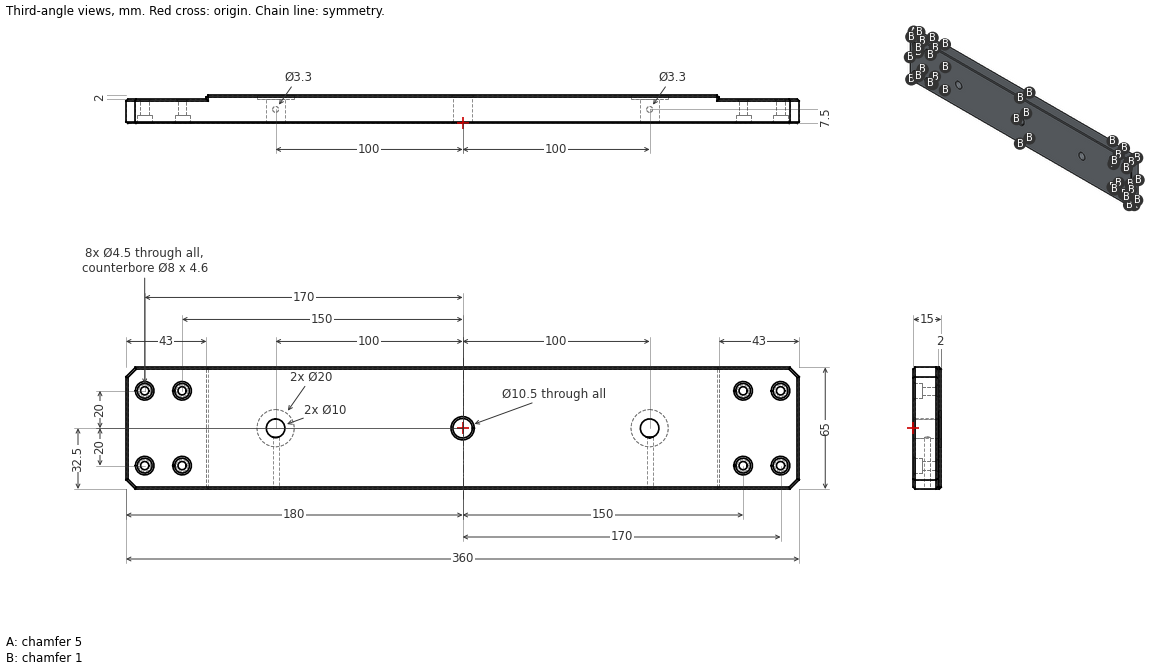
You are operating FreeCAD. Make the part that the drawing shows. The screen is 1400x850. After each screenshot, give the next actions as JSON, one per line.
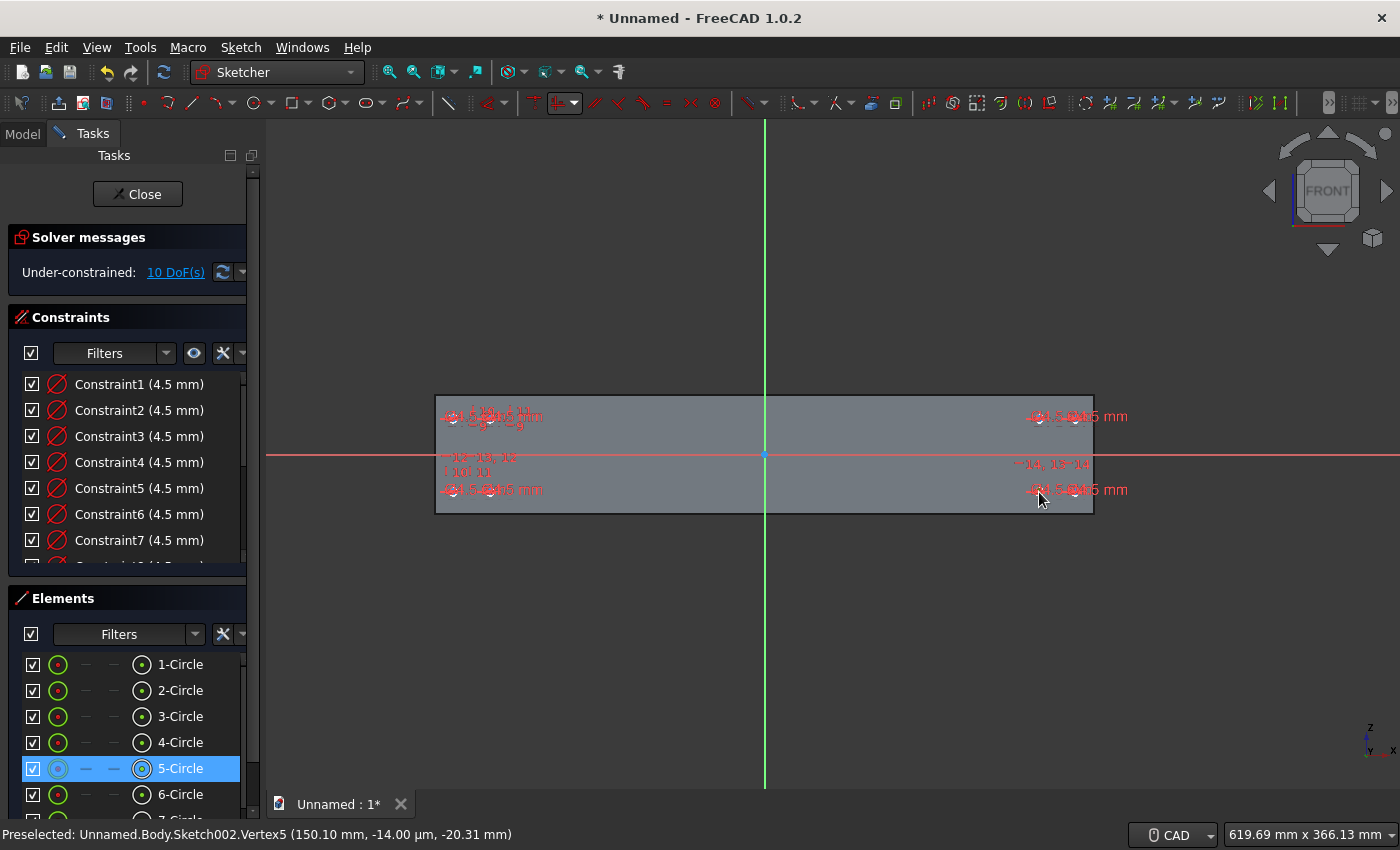
{"action": "left_click", "coordinate": [1039, 419]}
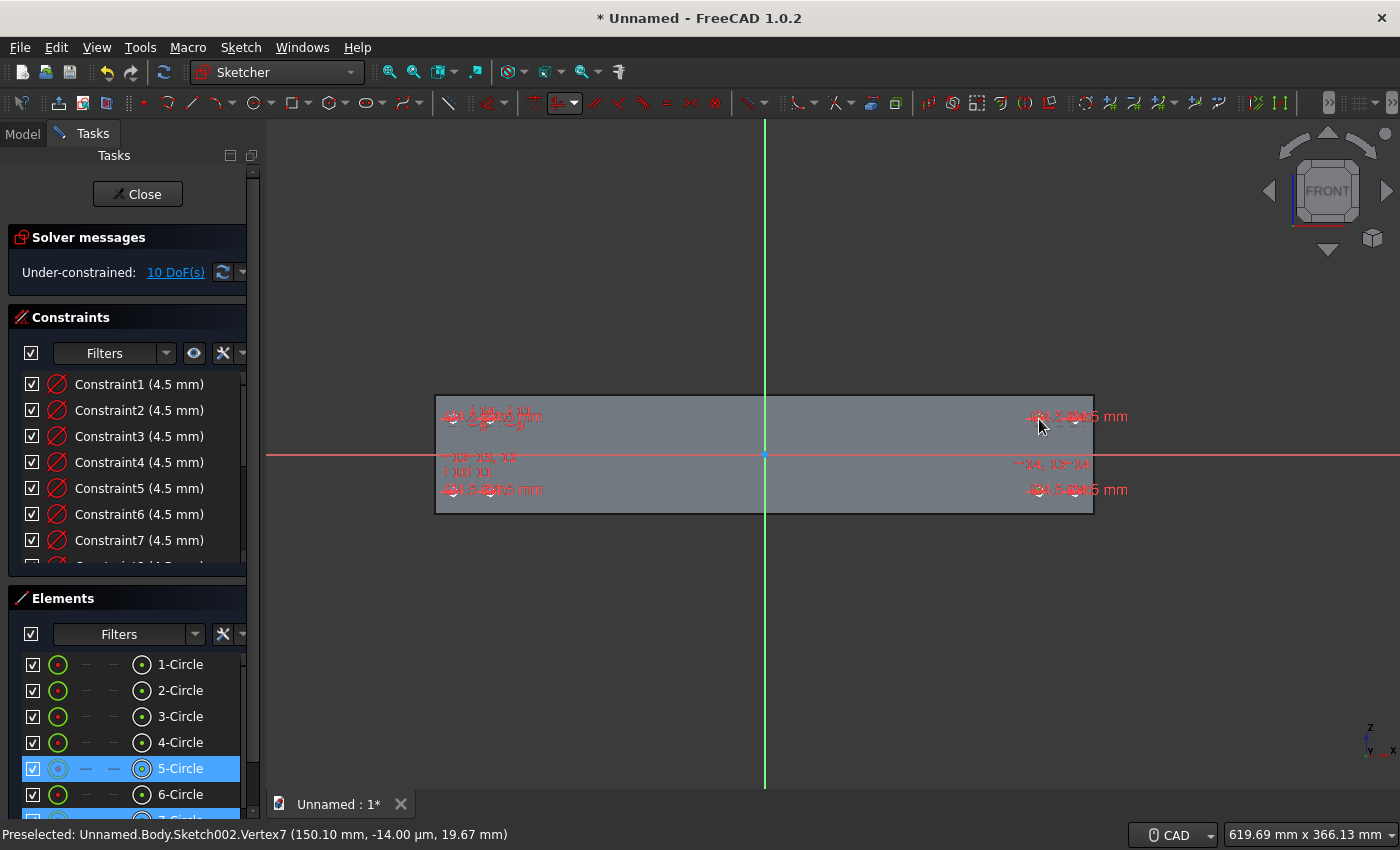
{"action": "key", "text": "v"}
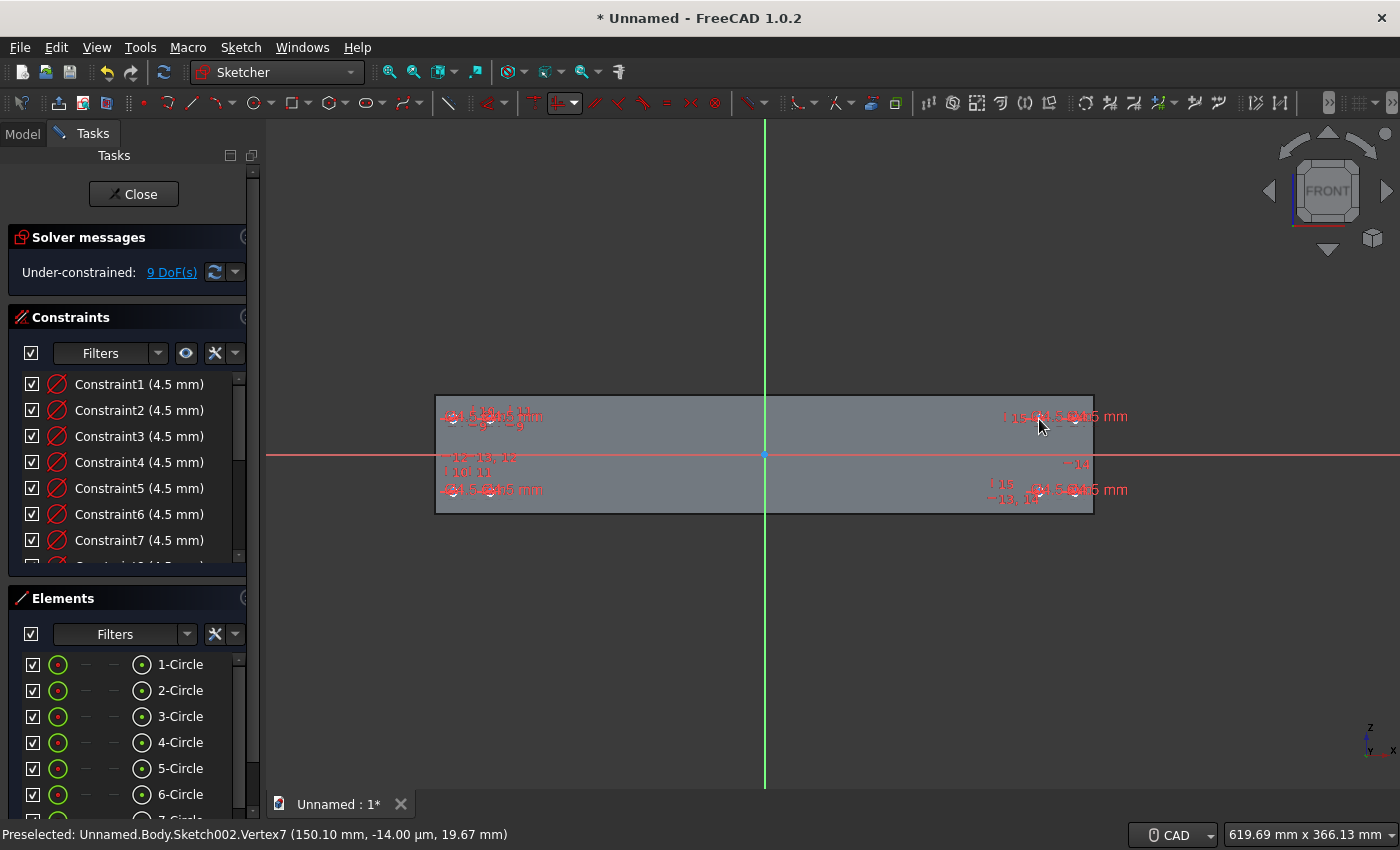
{"action": "left_click", "coordinate": [490, 419]}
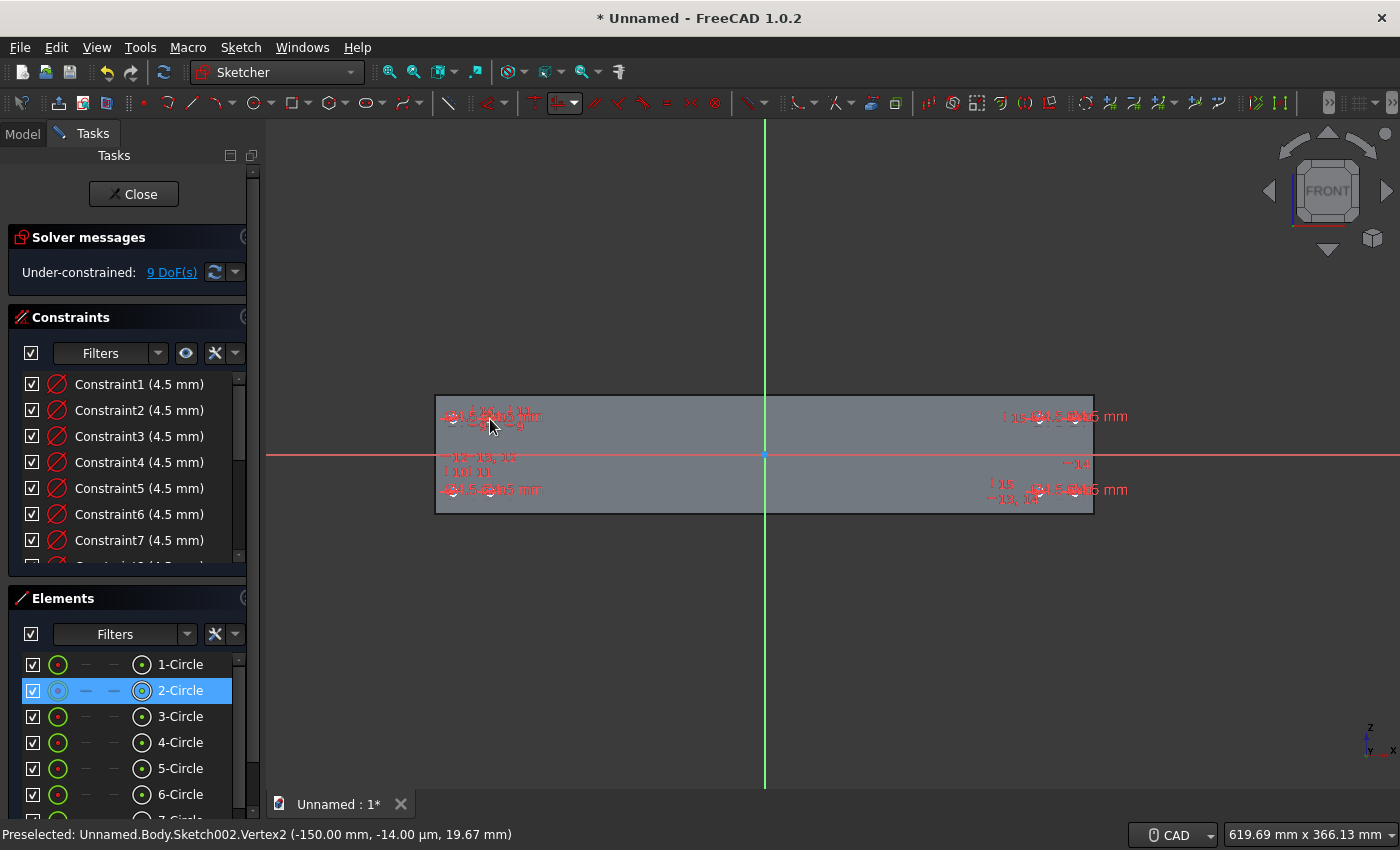
{"action": "left_click", "coordinate": [1039, 419]}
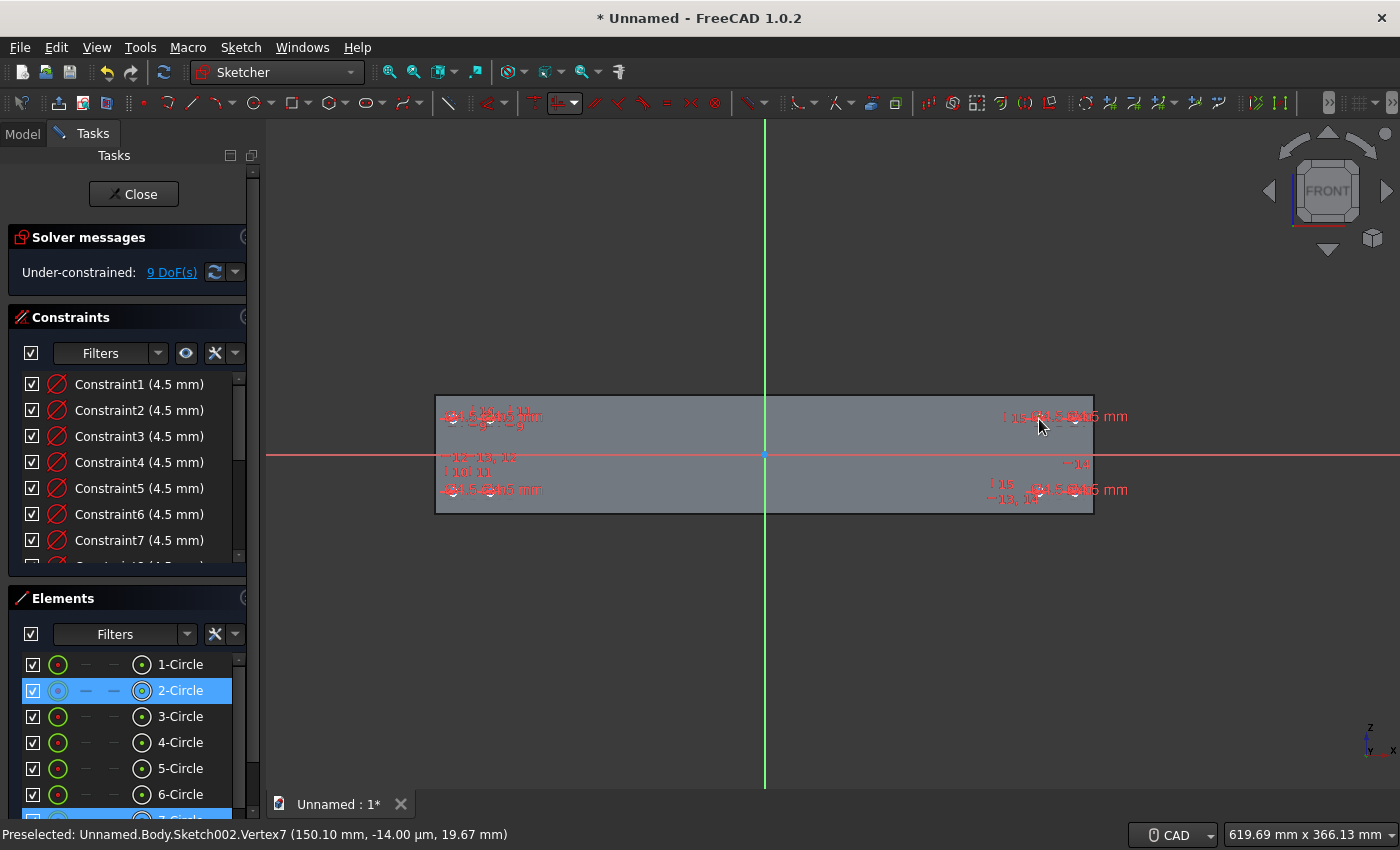
{"action": "left_click", "coordinate": [576, 104]}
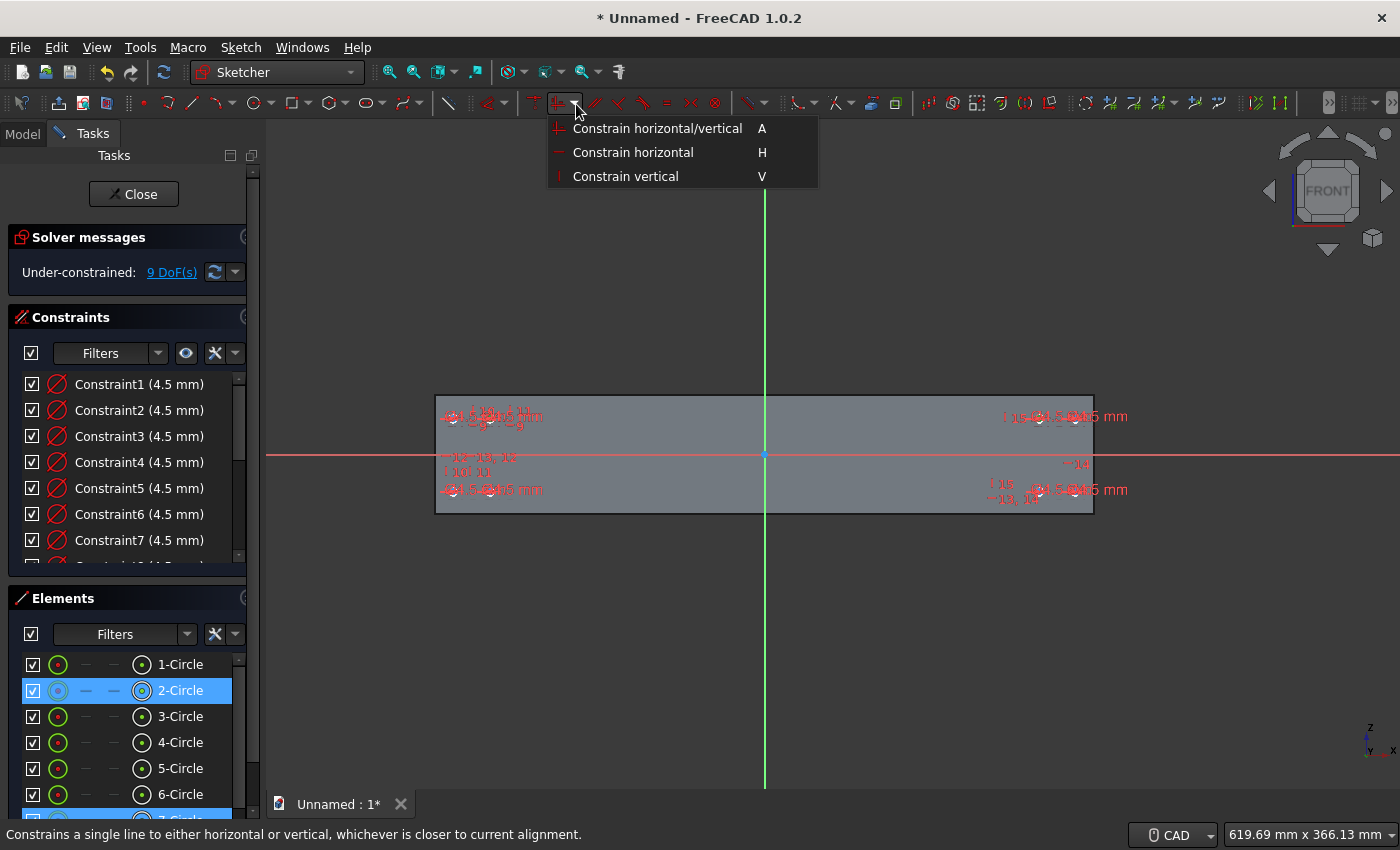
{"action": "left_click", "coordinate": [683, 152]}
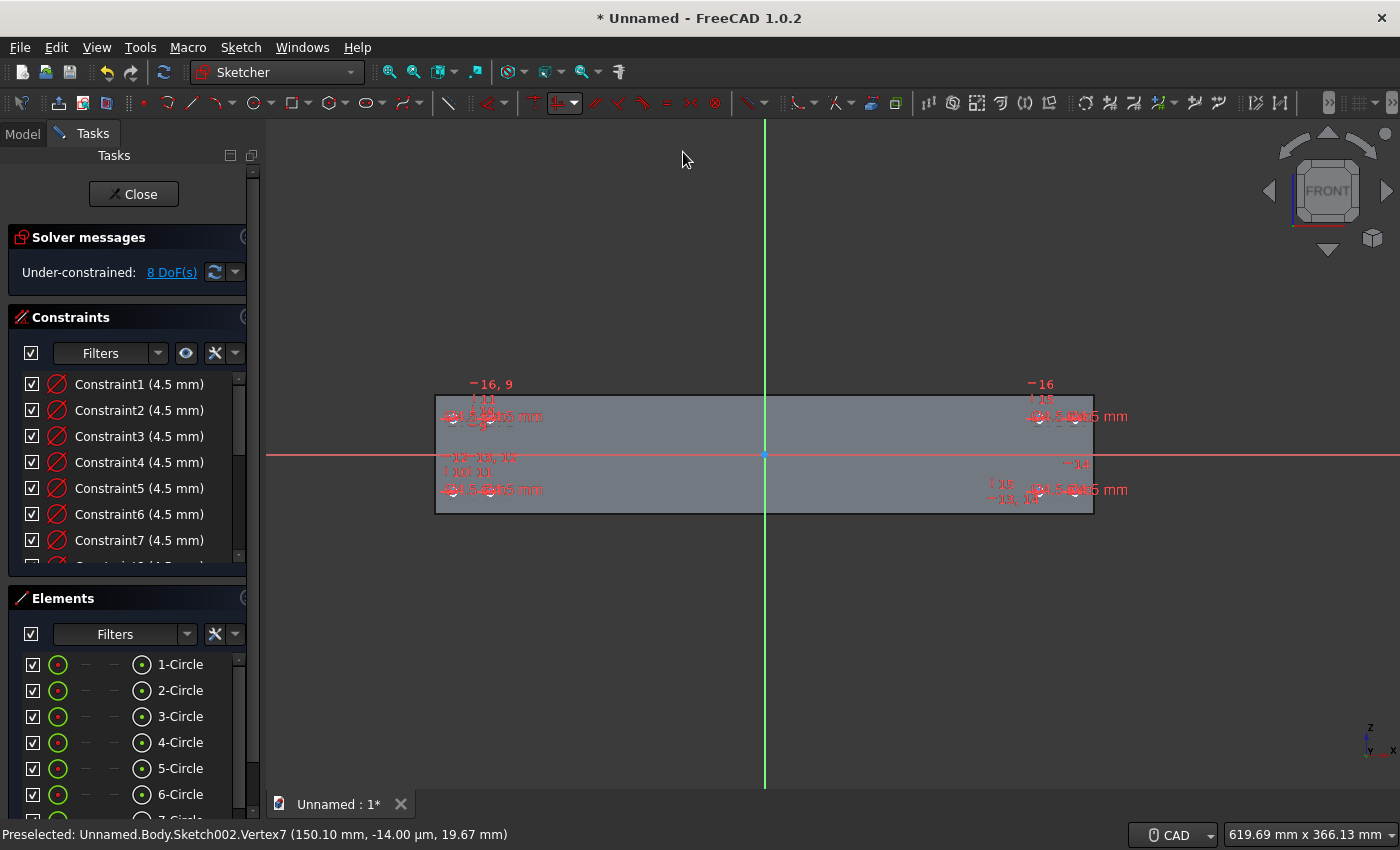
{"action": "left_click", "coordinate": [1075, 492]}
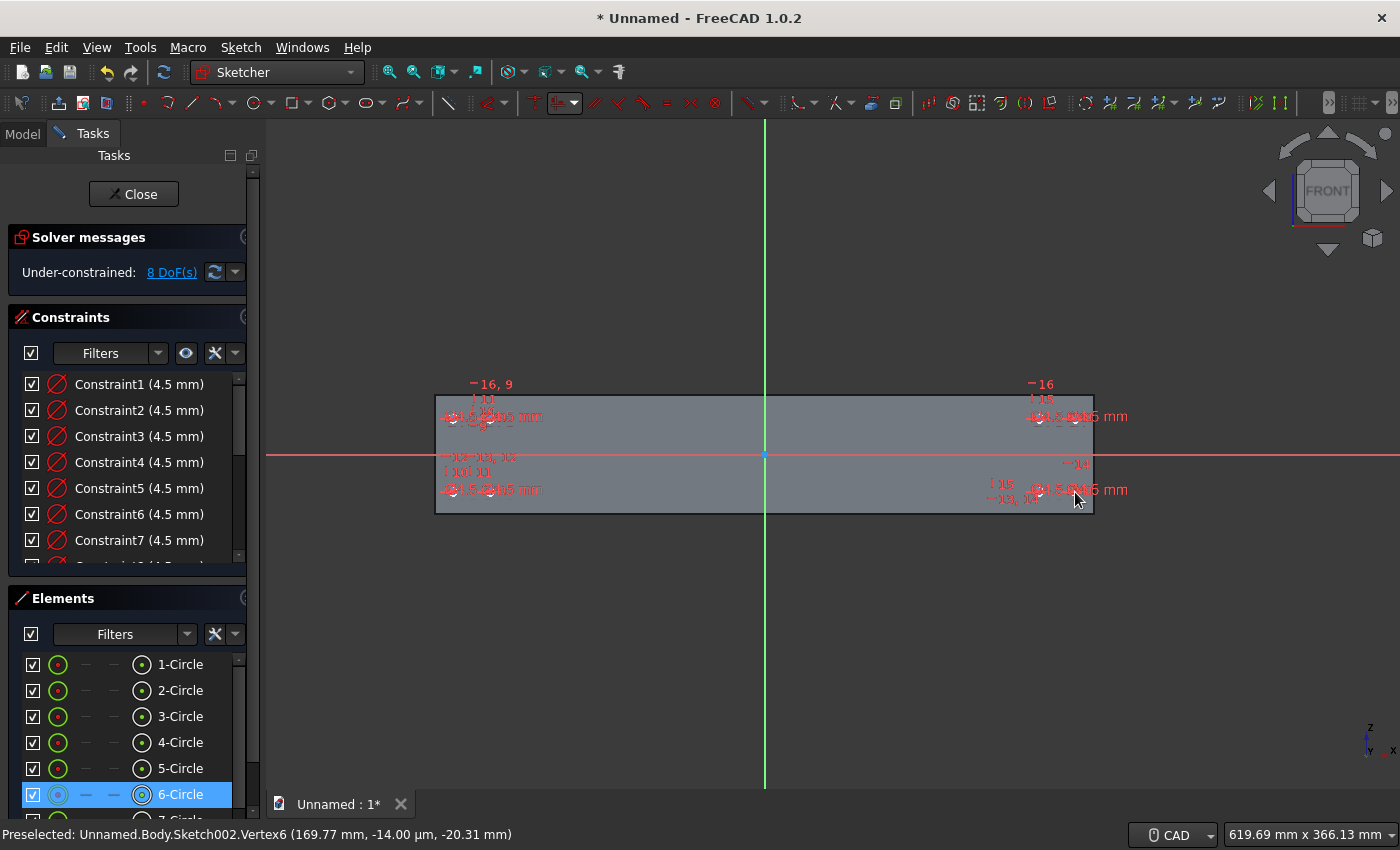
{"action": "left_click", "coordinate": [1075, 419]}